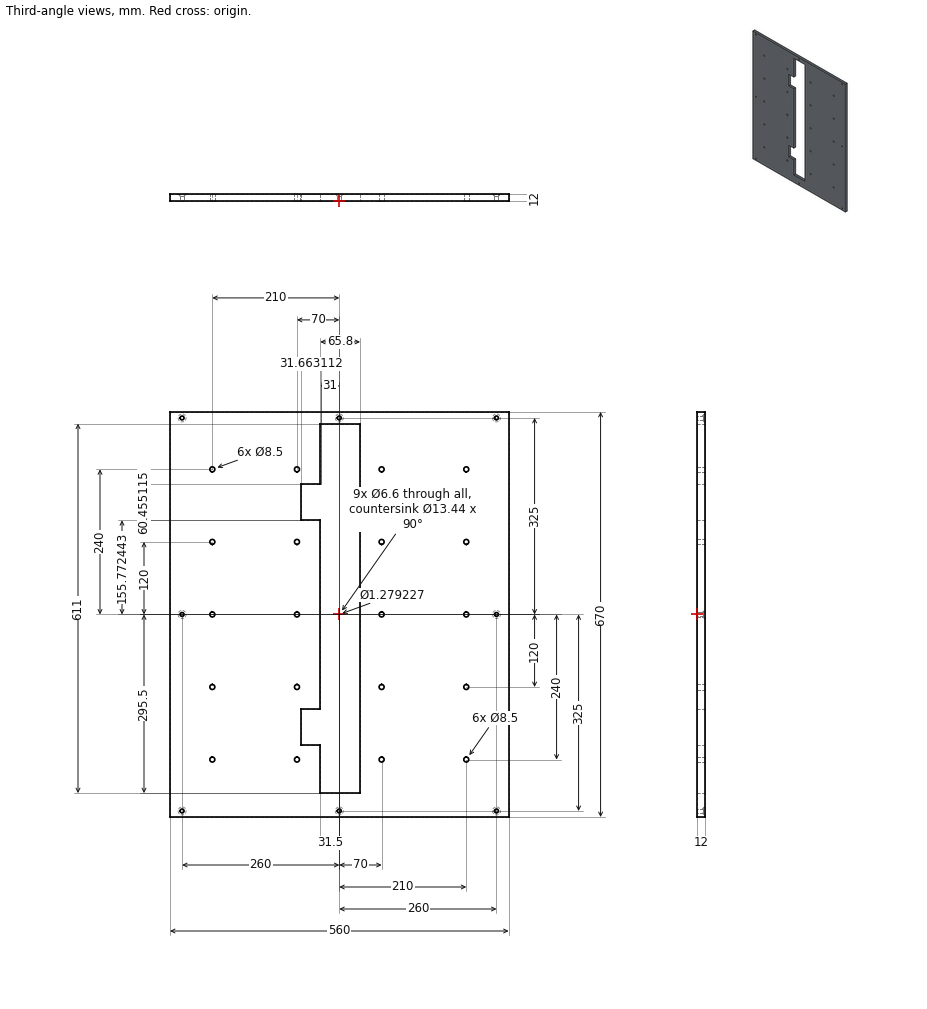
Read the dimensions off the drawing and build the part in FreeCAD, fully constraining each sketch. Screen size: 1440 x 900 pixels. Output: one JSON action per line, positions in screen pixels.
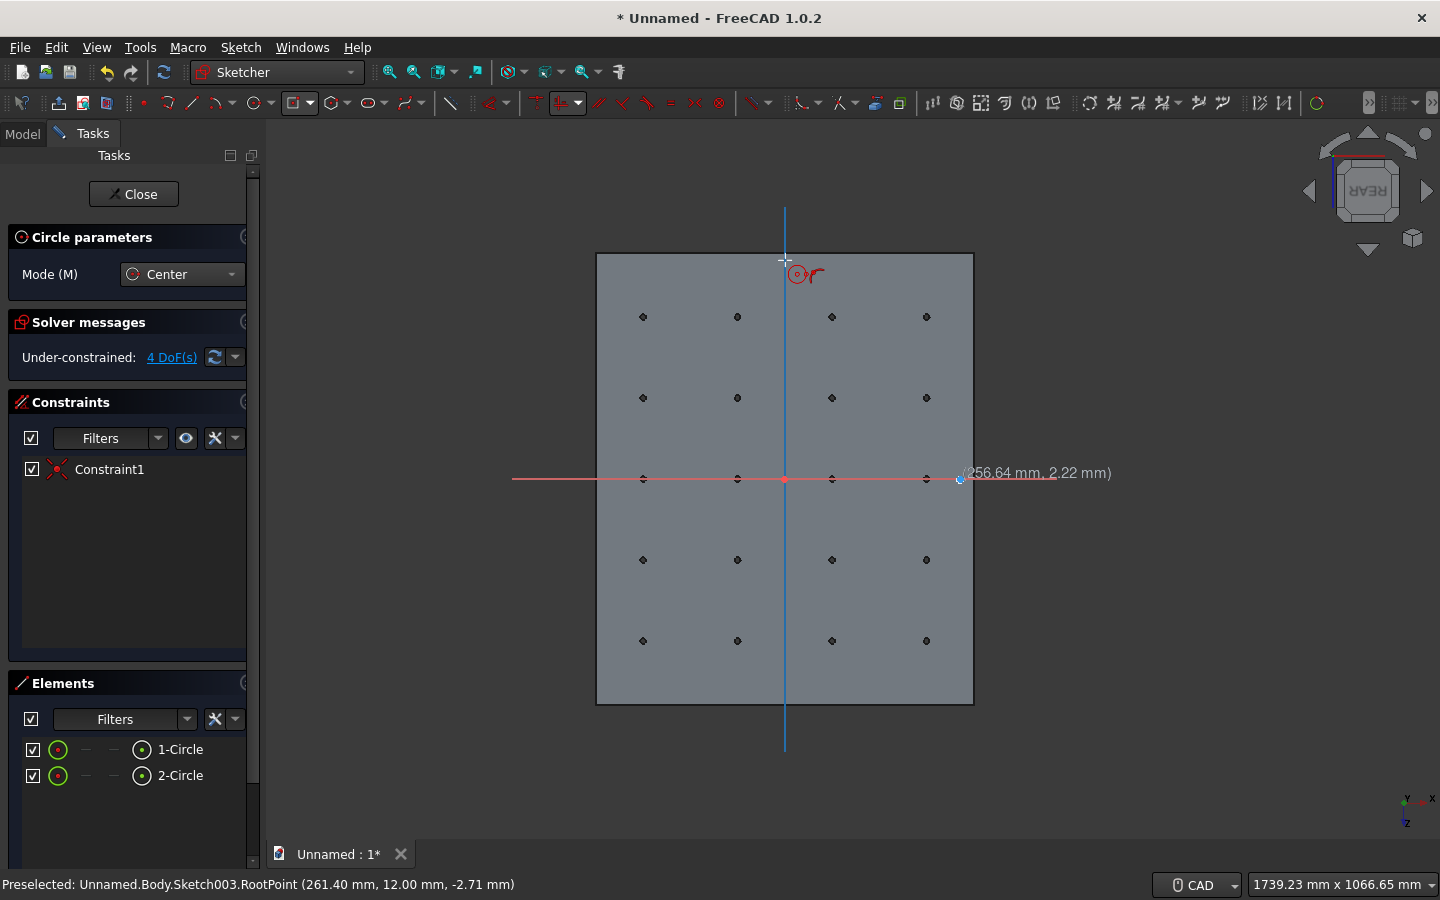
{"action": "left_click", "coordinate": [785, 260]}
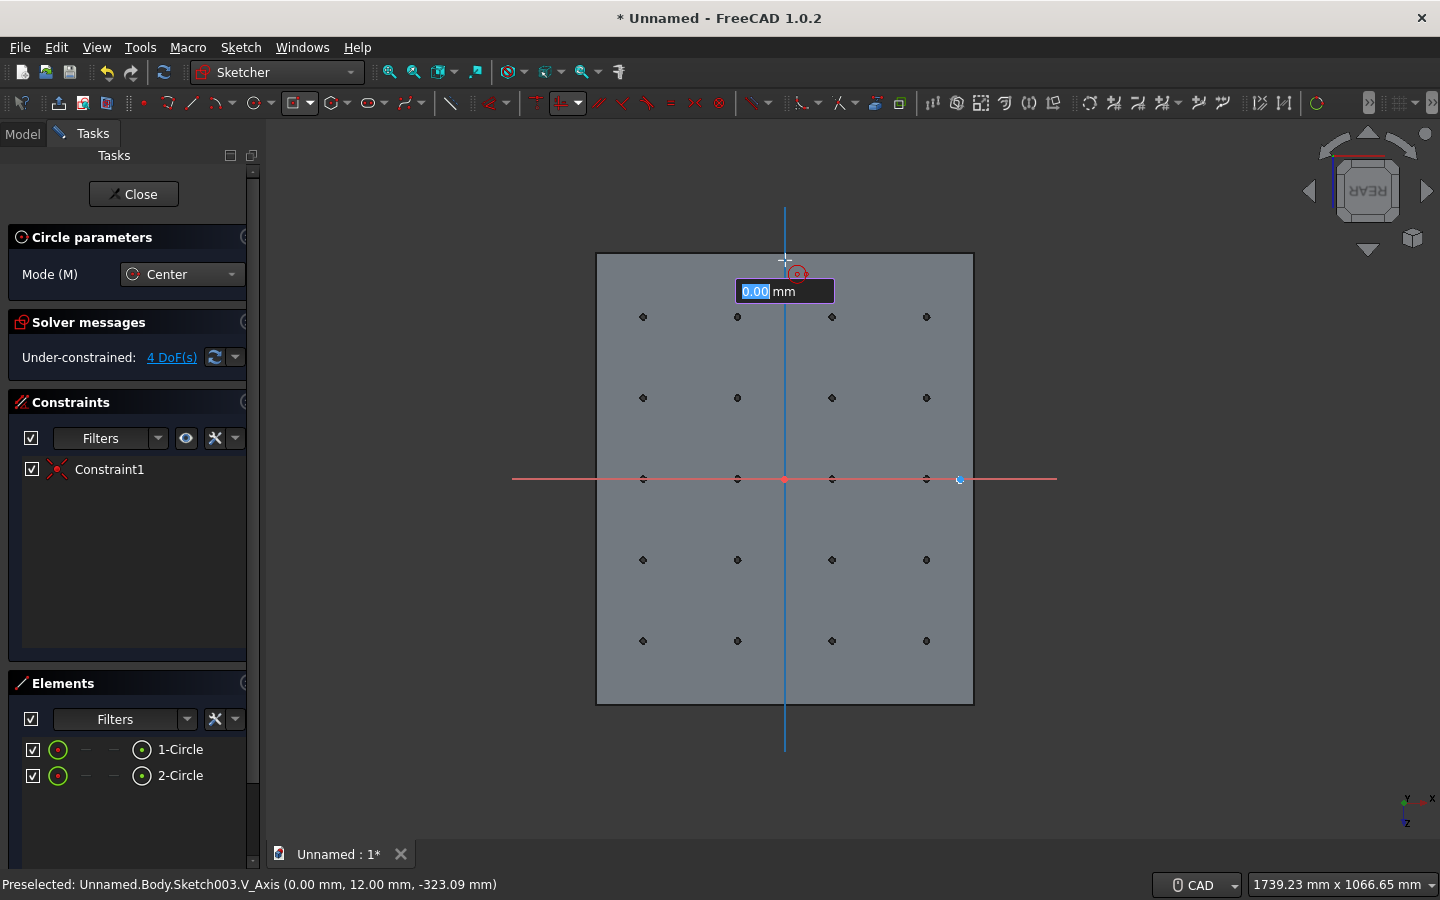
{"action": "scroll", "coordinate": [787, 259], "scroll_direction": "up", "scroll_amount": 11}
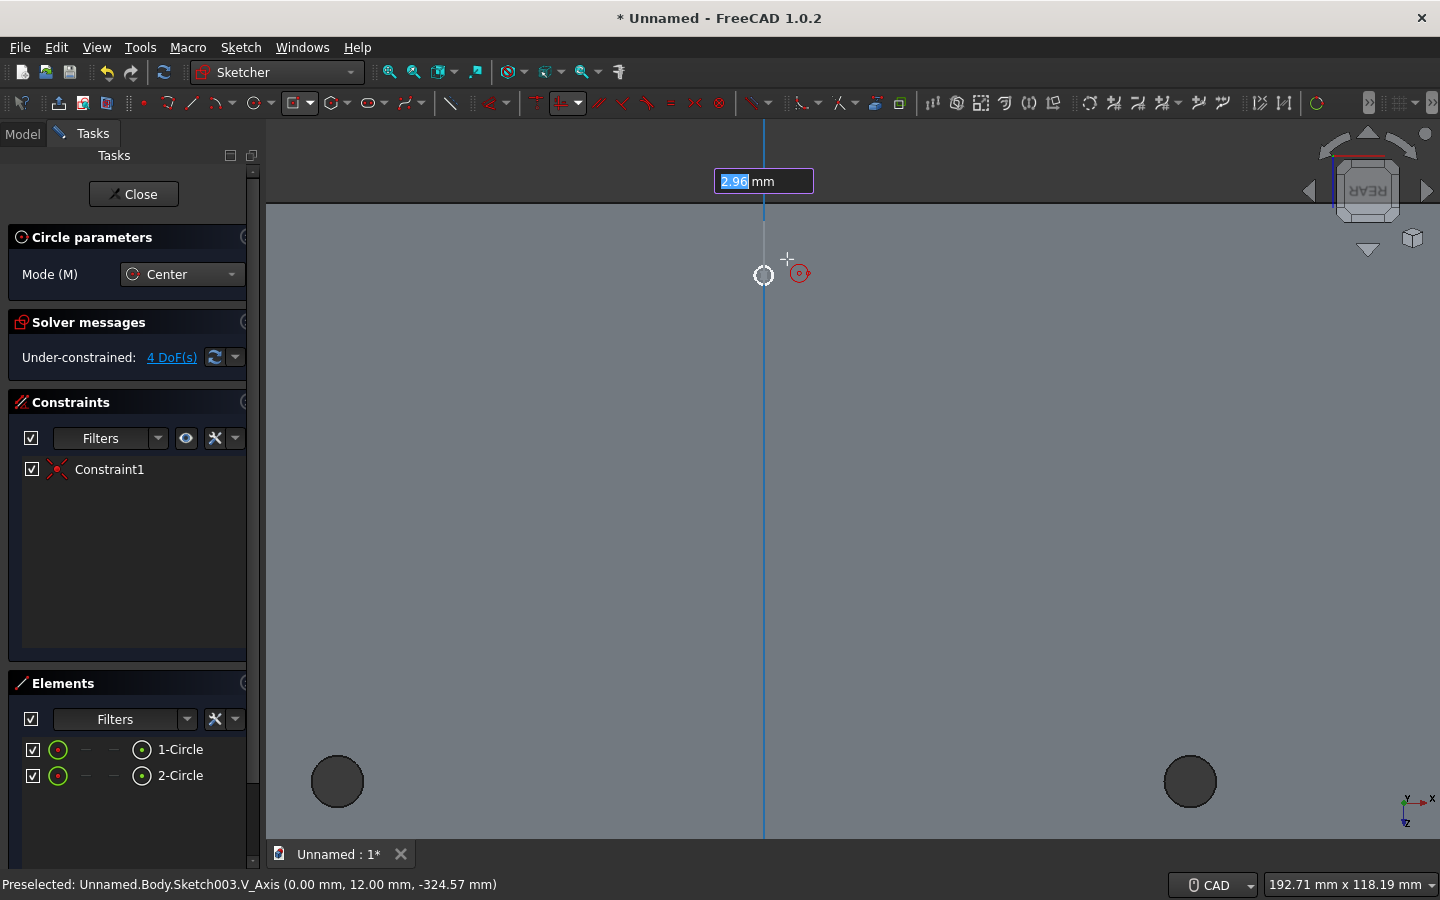
{"action": "left_click", "coordinate": [783, 257]}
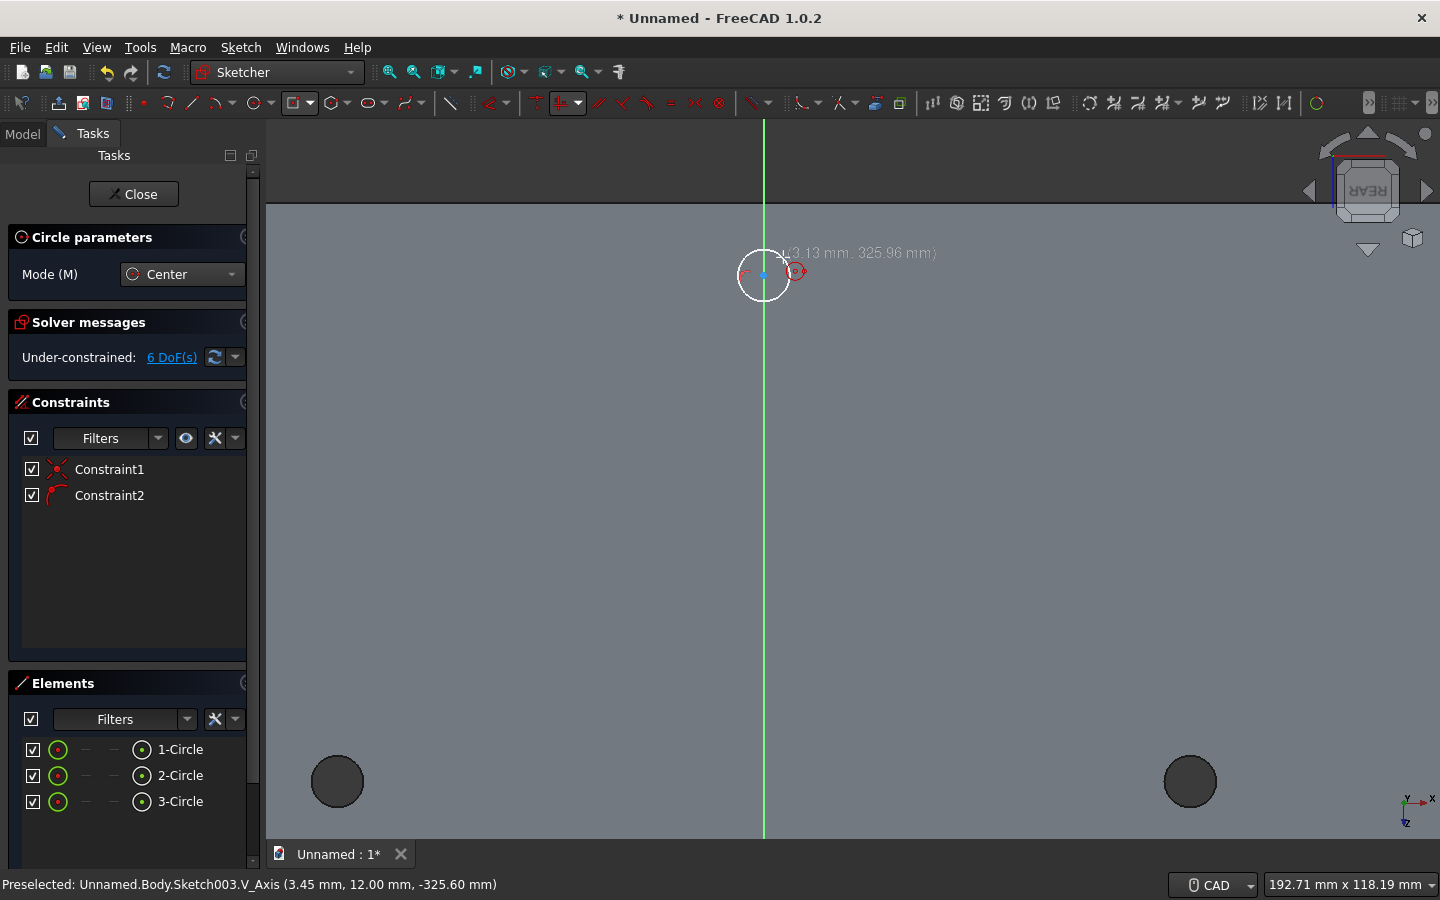
{"action": "scroll", "coordinate": [787, 259], "scroll_direction": "down", "scroll_amount": 11}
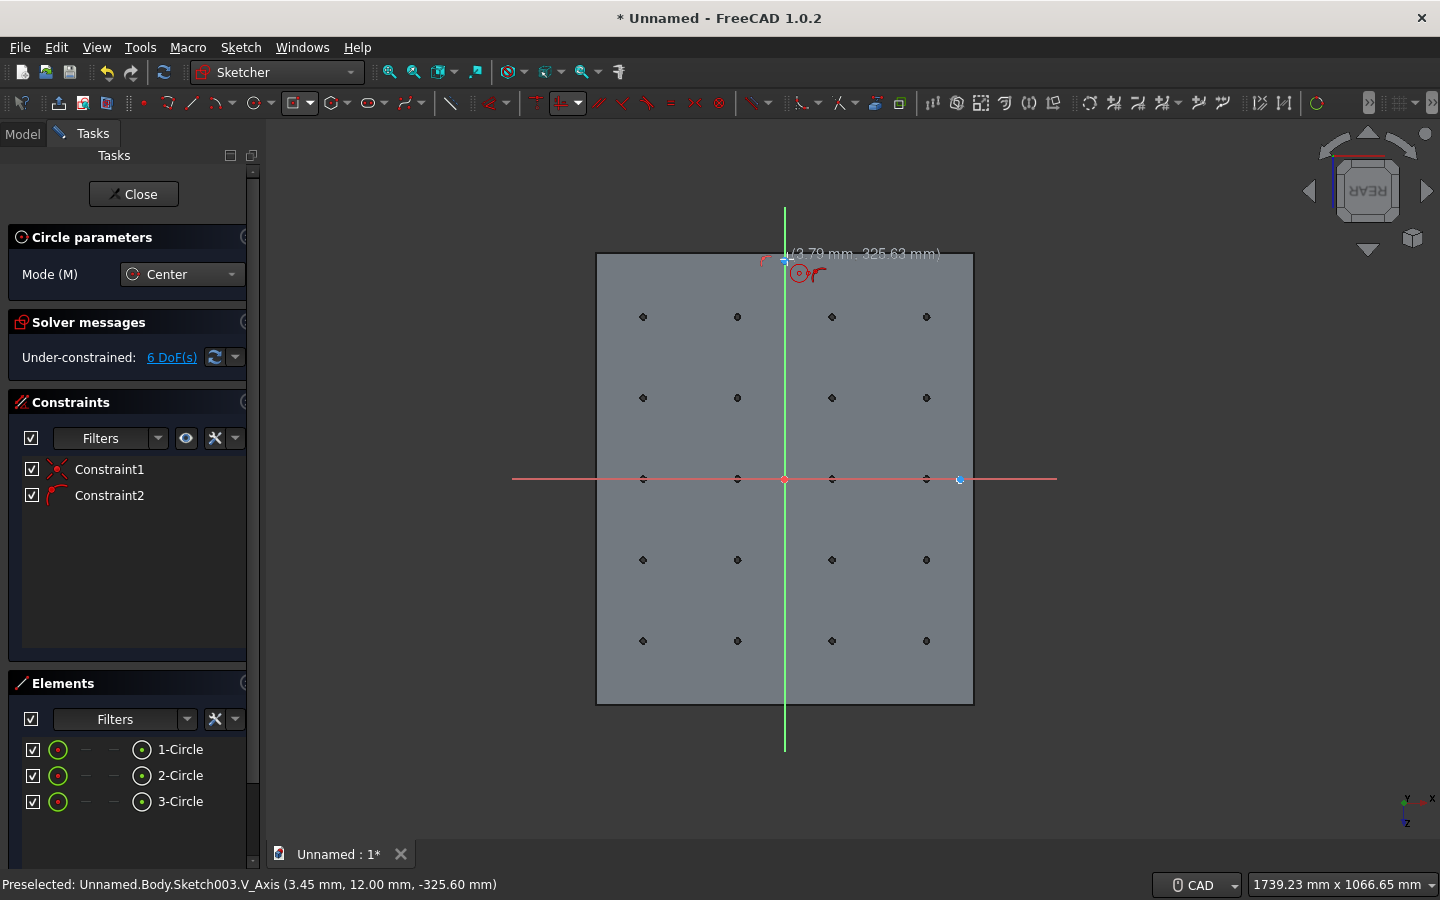
{"action": "scroll", "coordinate": [960, 260], "scroll_direction": "up", "scroll_amount": 12}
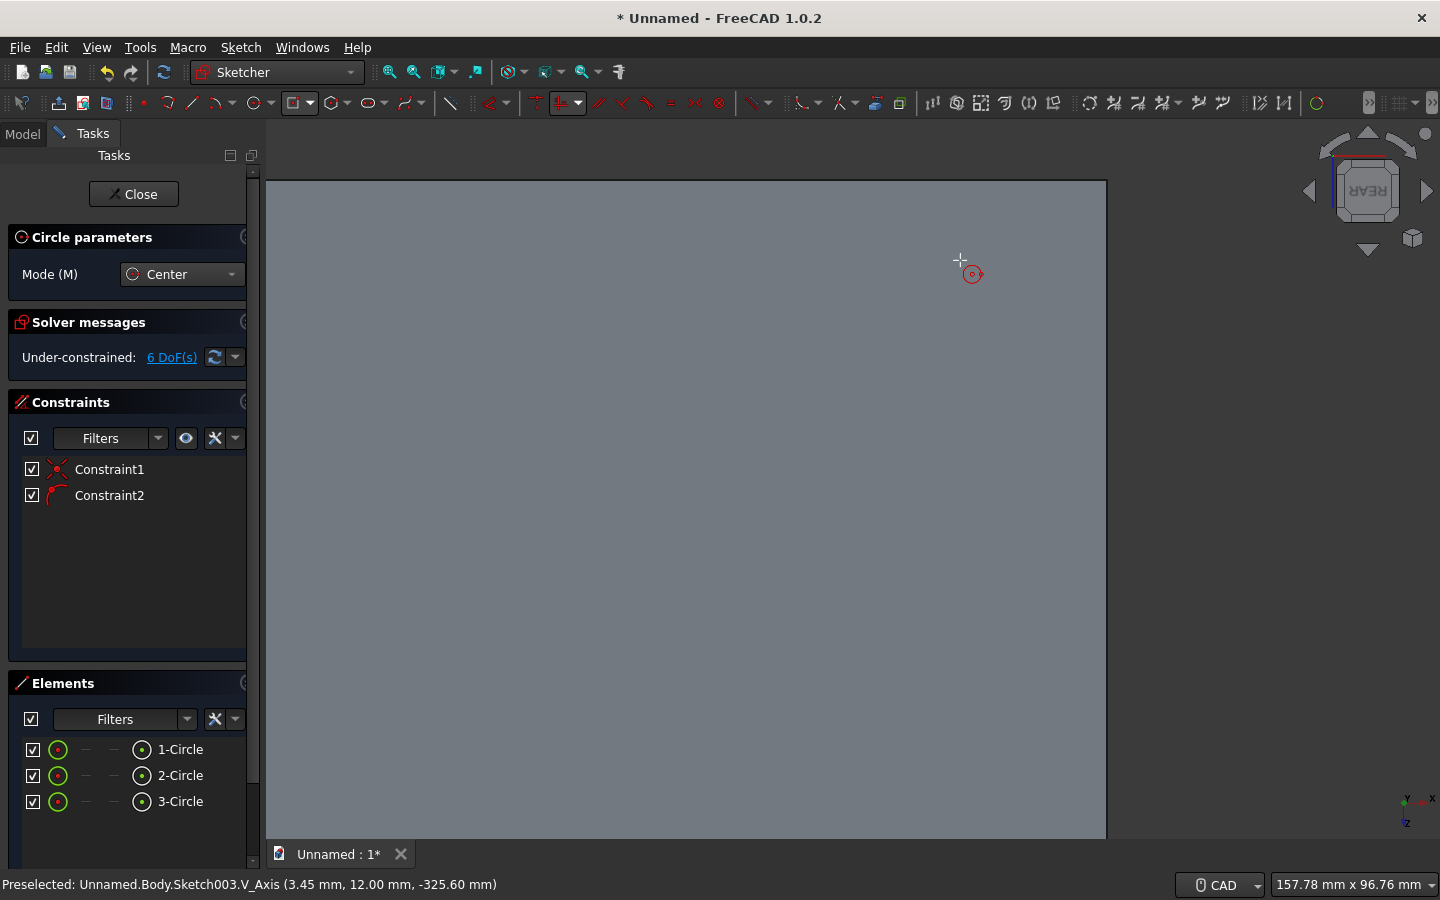
{"action": "scroll", "coordinate": [960, 260], "scroll_direction": "down", "scroll_amount": 12}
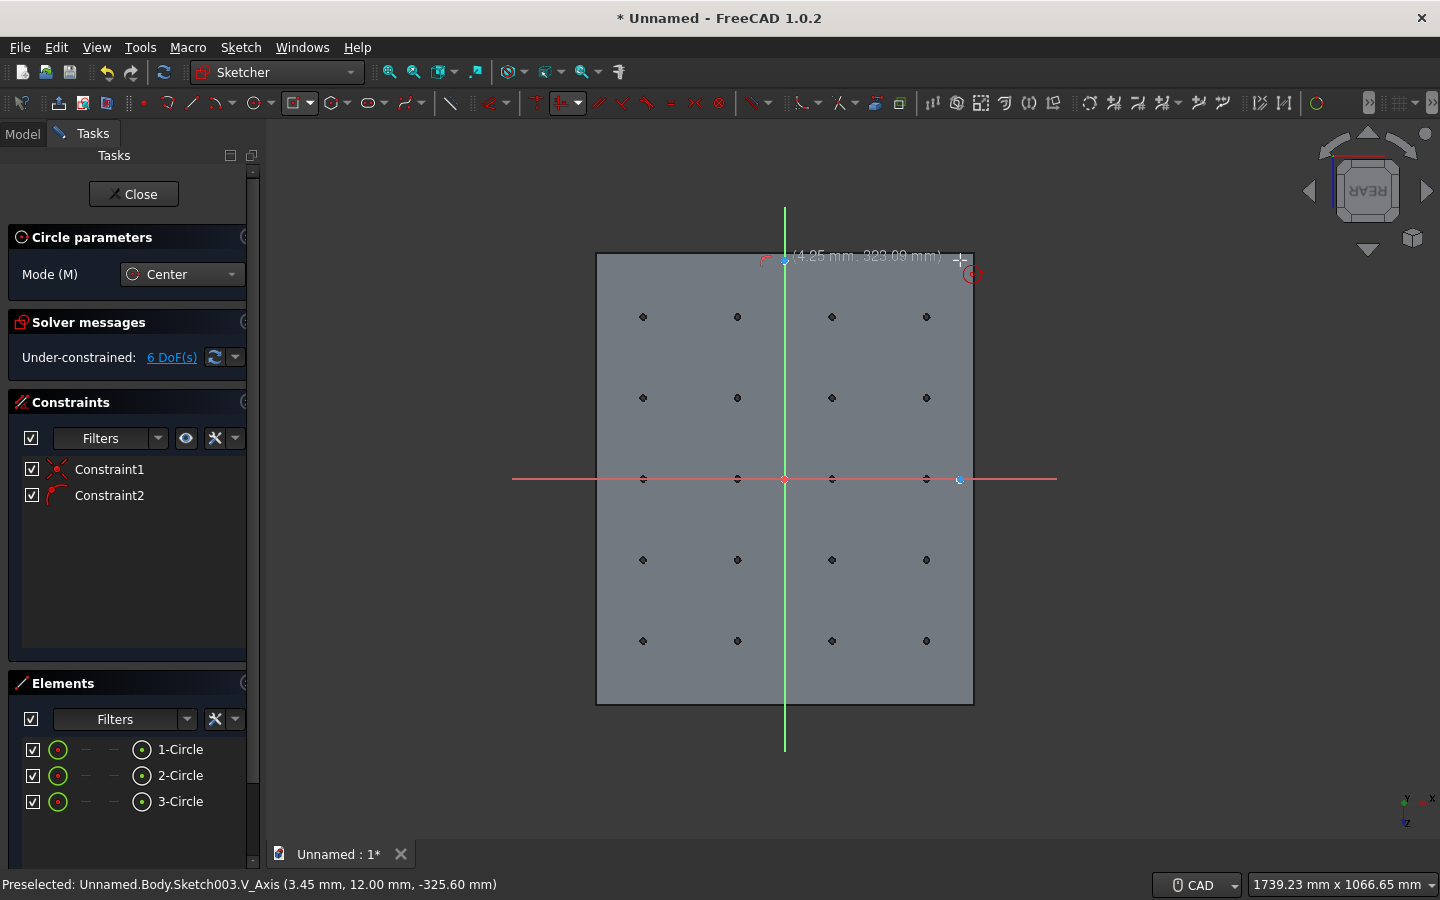
{"action": "left_click", "coordinate": [960, 260]}